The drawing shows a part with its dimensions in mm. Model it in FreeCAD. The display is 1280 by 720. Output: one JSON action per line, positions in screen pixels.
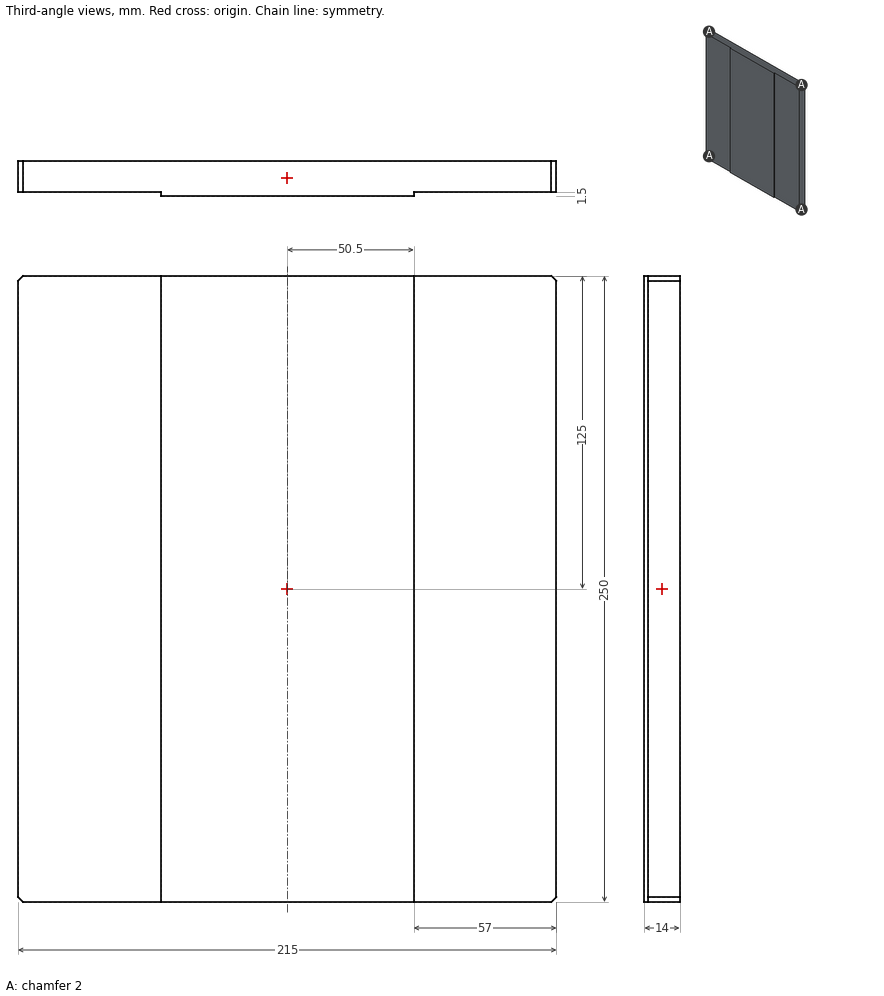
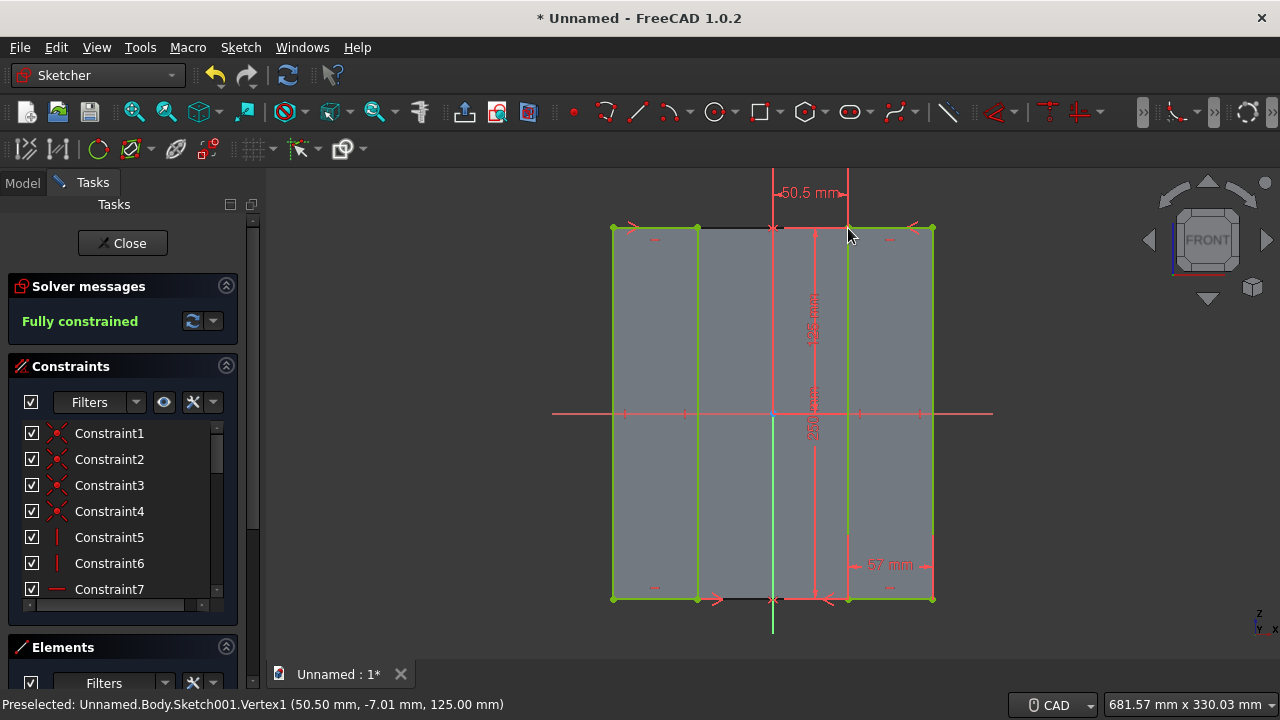
{"action": "left_click", "coordinate": [123, 243]}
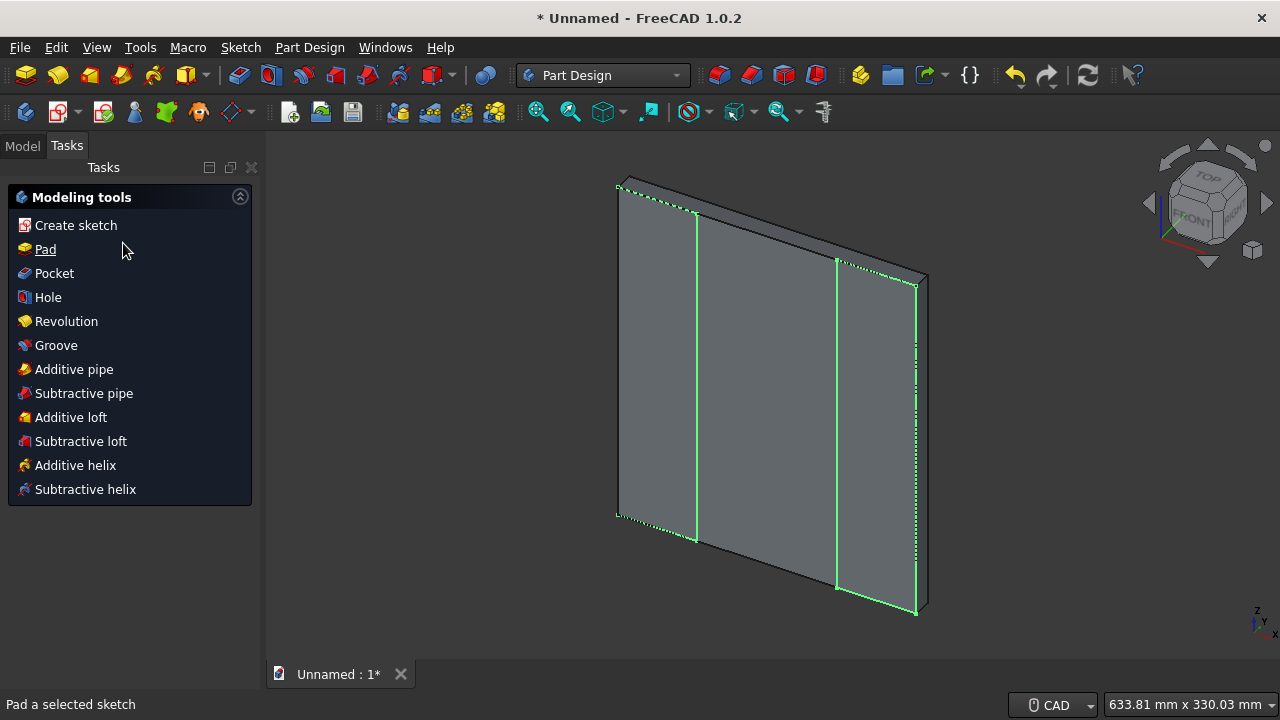
{"action": "left_click", "coordinate": [240, 76]}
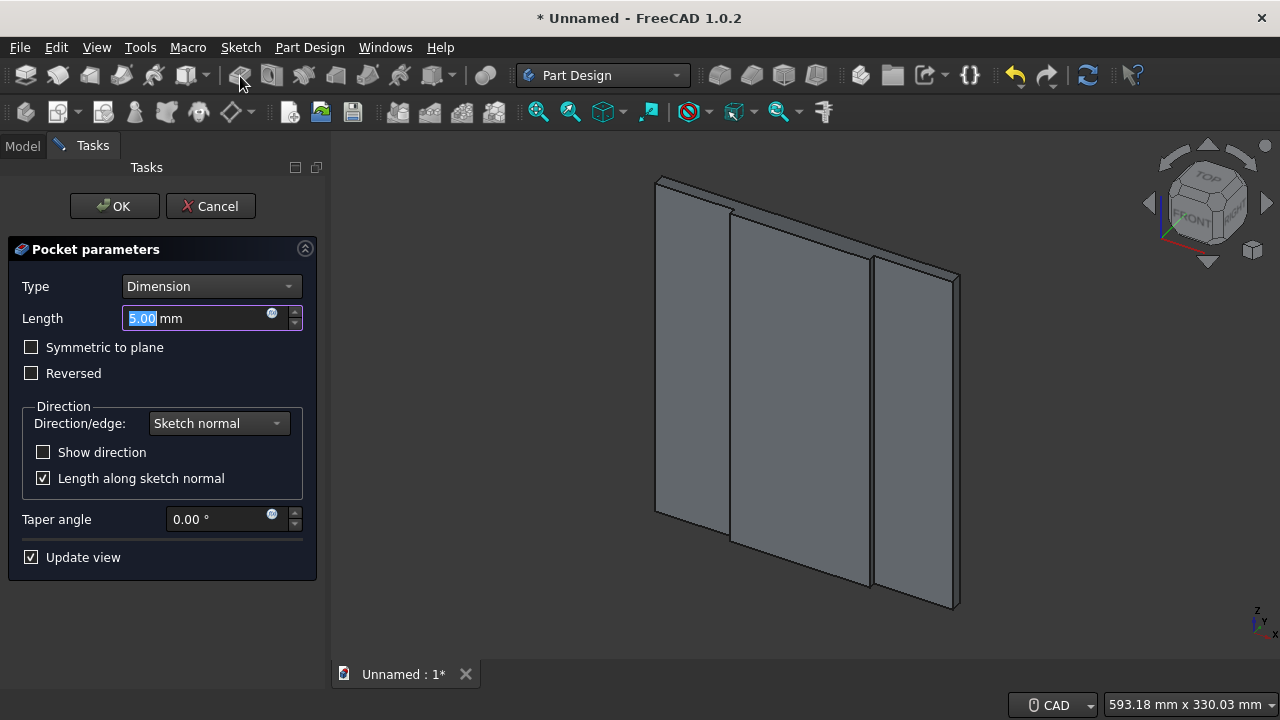
{"action": "type", "text": "1.5"}
{"action": "key", "text": "Tab"}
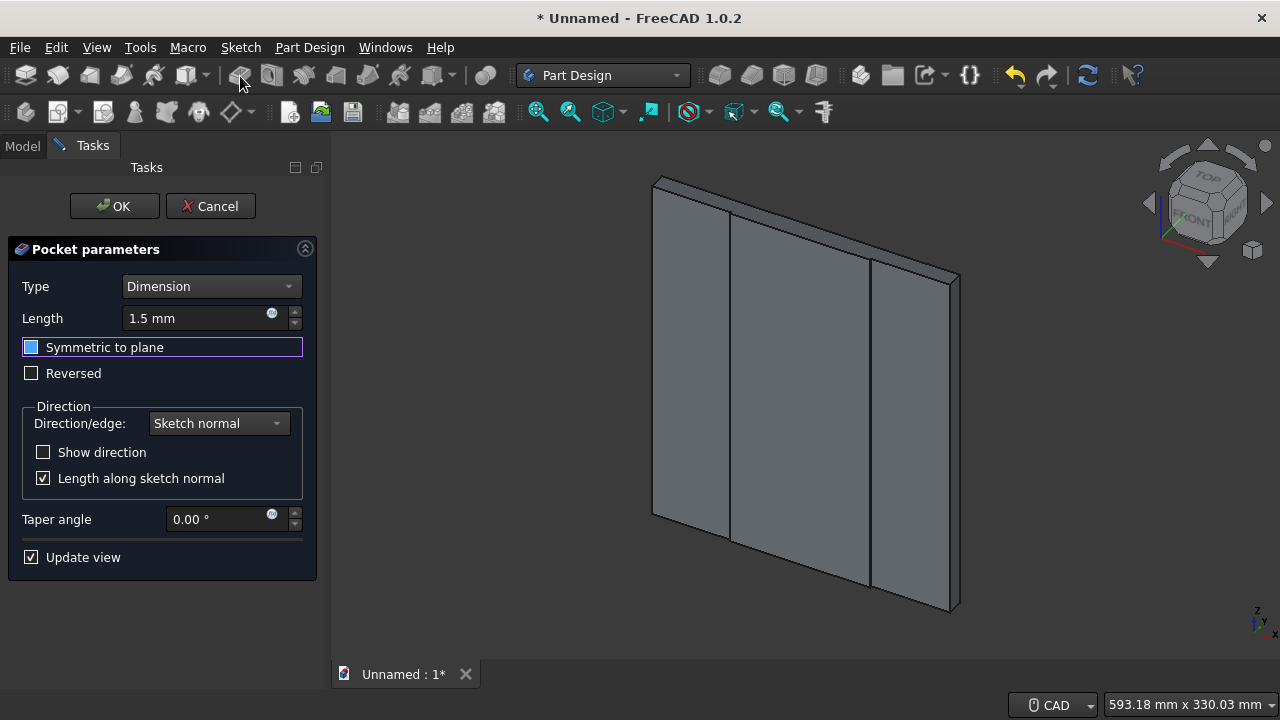
{"action": "left_click", "coordinate": [115, 206]}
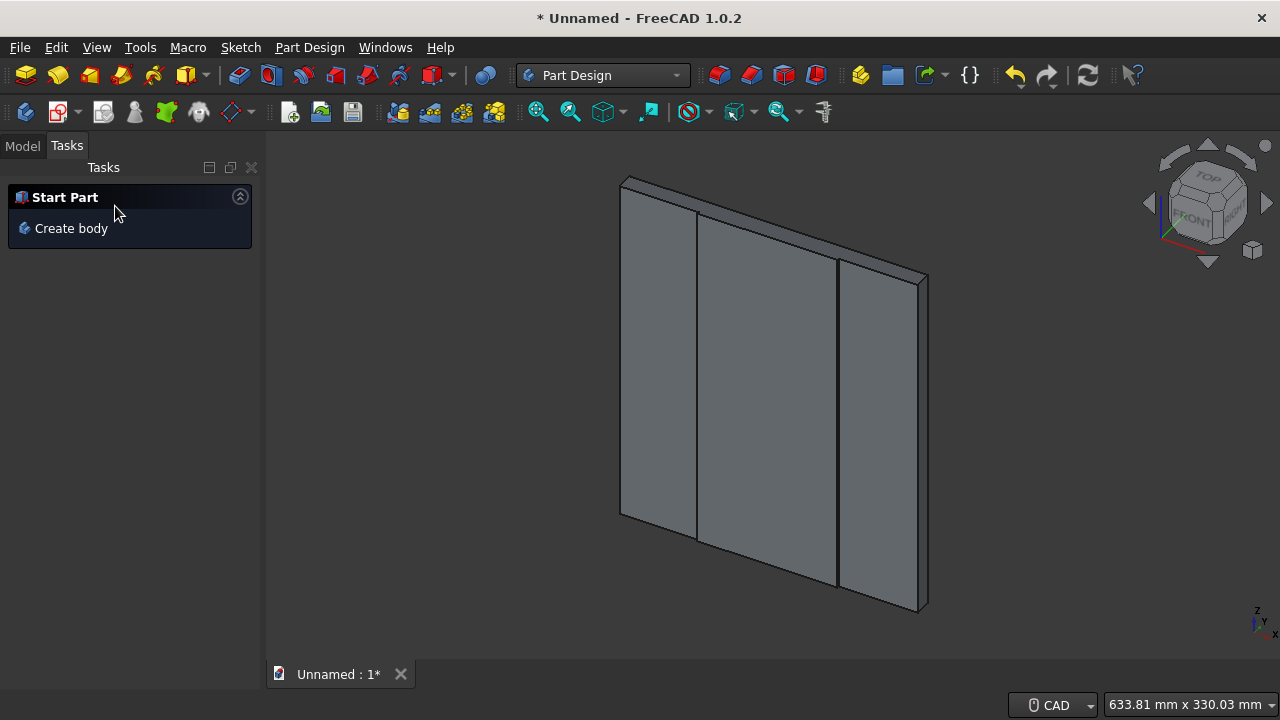
{"action": "left_click", "coordinate": [923, 279]}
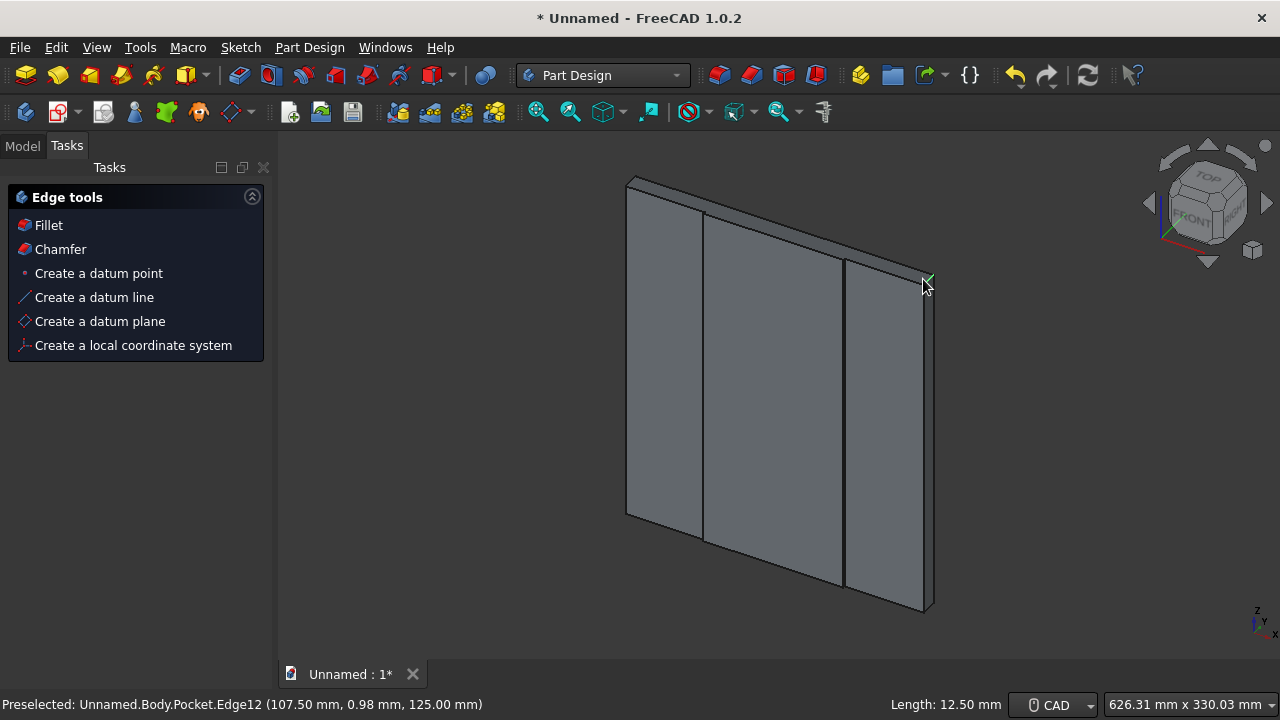
{"action": "scroll", "coordinate": [631, 180], "scroll_direction": "up", "scroll_amount": 4}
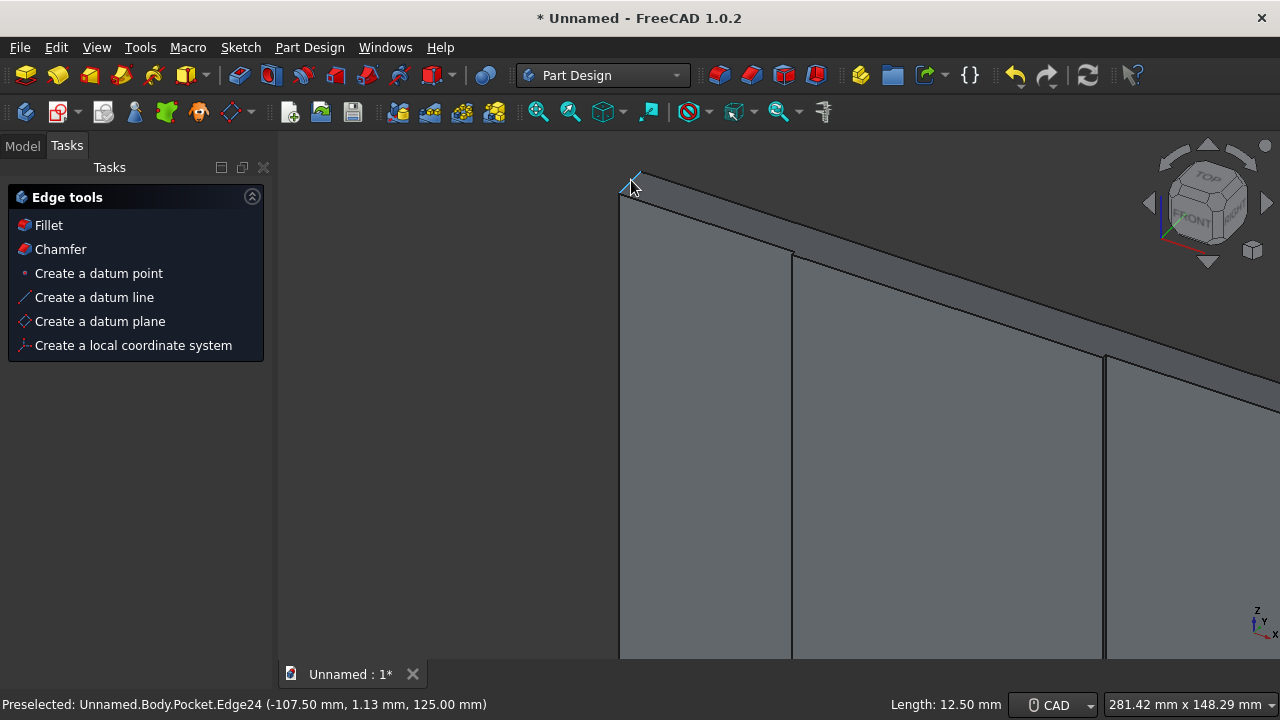
{"action": "left_click", "coordinate": [540, 112]}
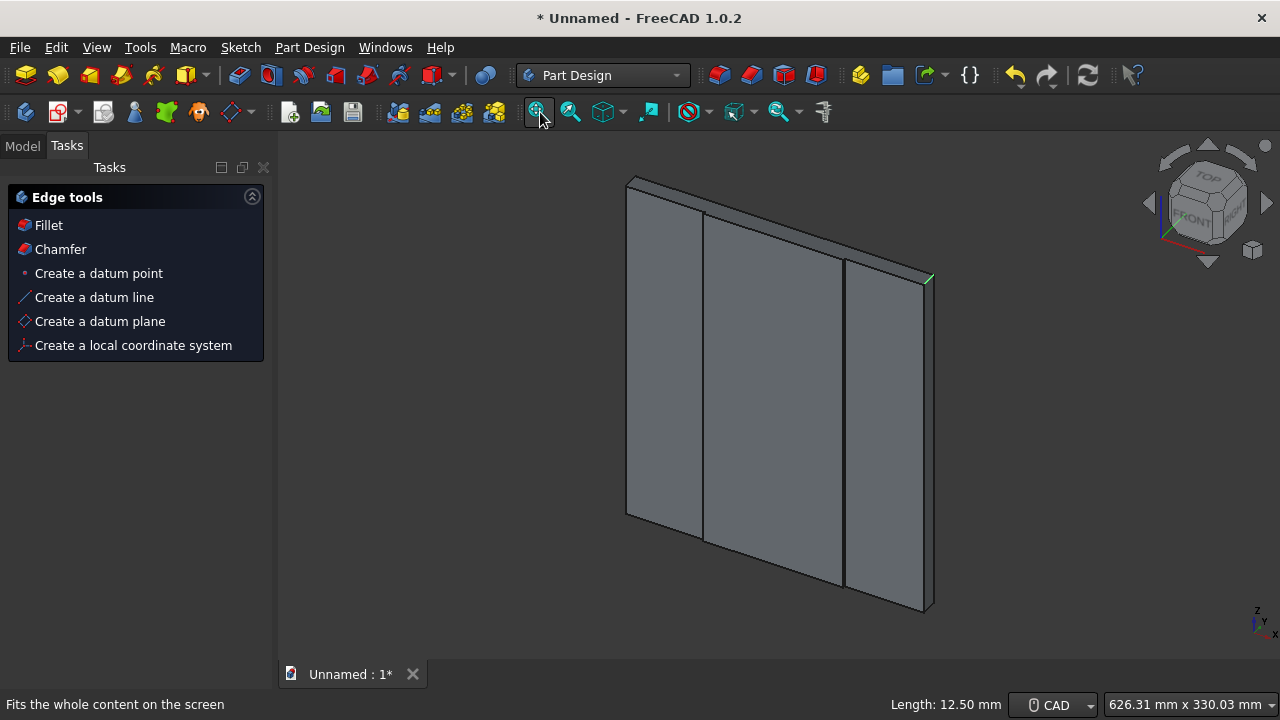
{"action": "key", "text": "0"}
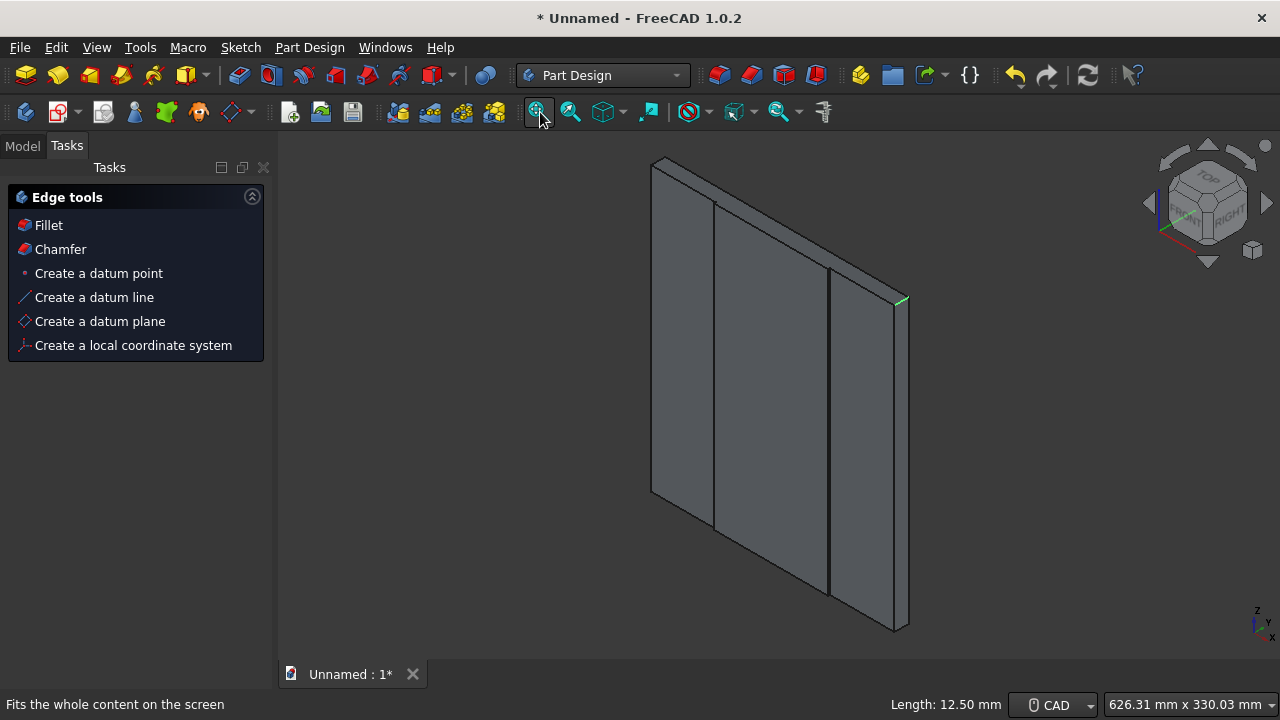
{"action": "scroll", "coordinate": [658, 160], "scroll_direction": "up", "scroll_amount": 4}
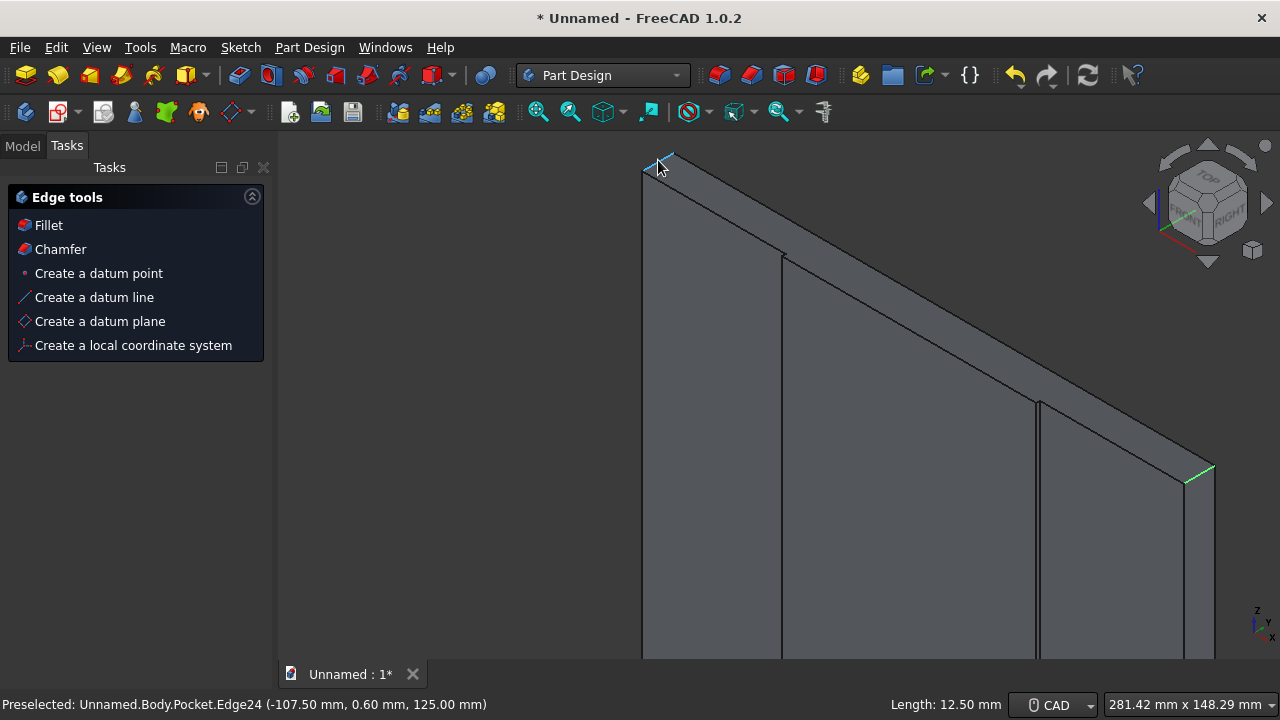
{"action": "key", "text": "v f"}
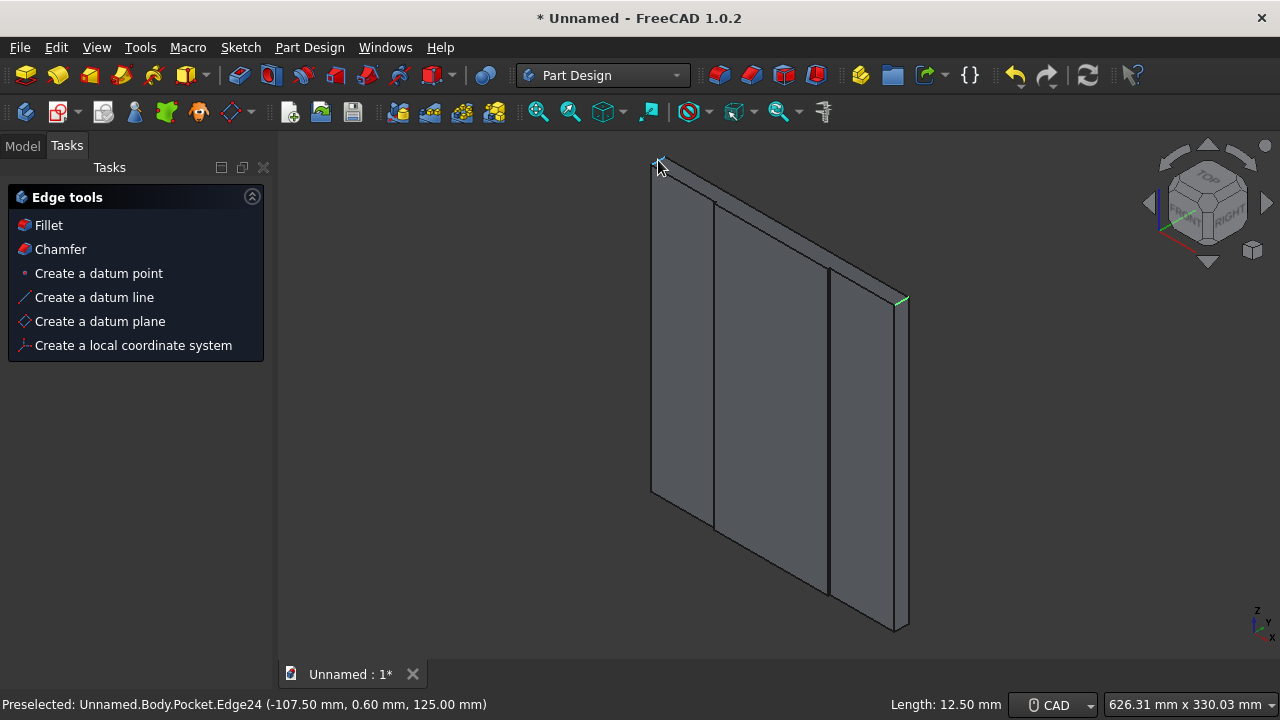
{"action": "key", "text": "2"}